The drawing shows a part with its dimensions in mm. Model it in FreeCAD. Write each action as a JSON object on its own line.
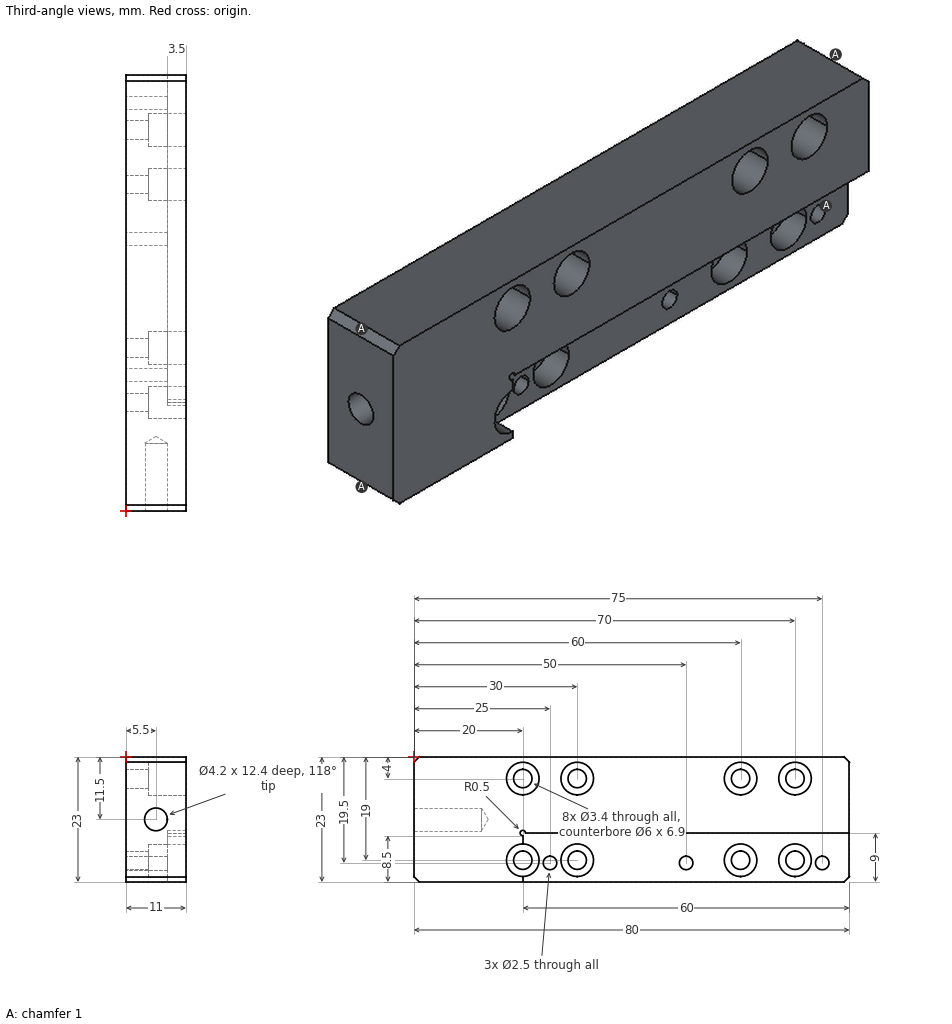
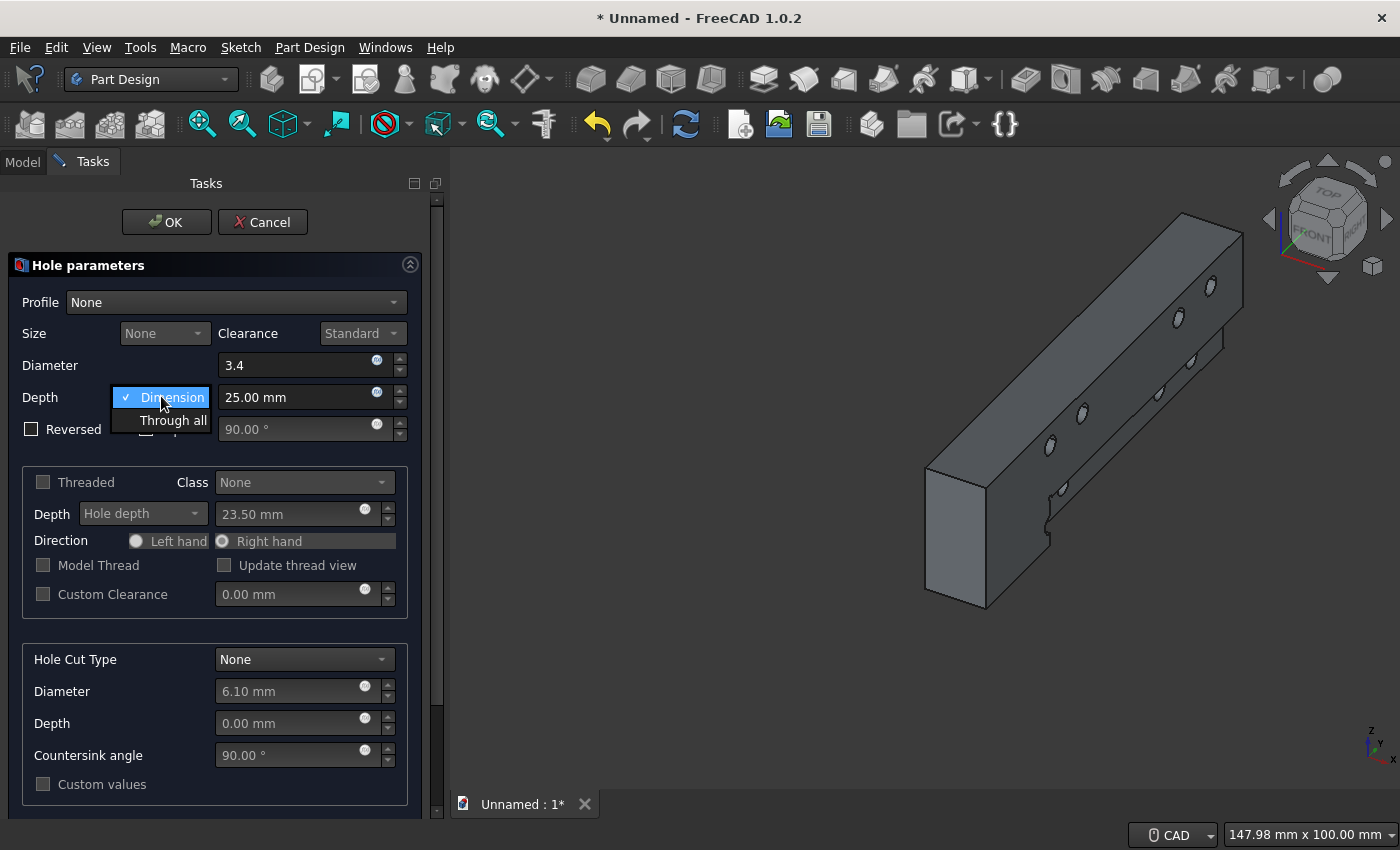
{"action": "left_click", "coordinate": [160, 420]}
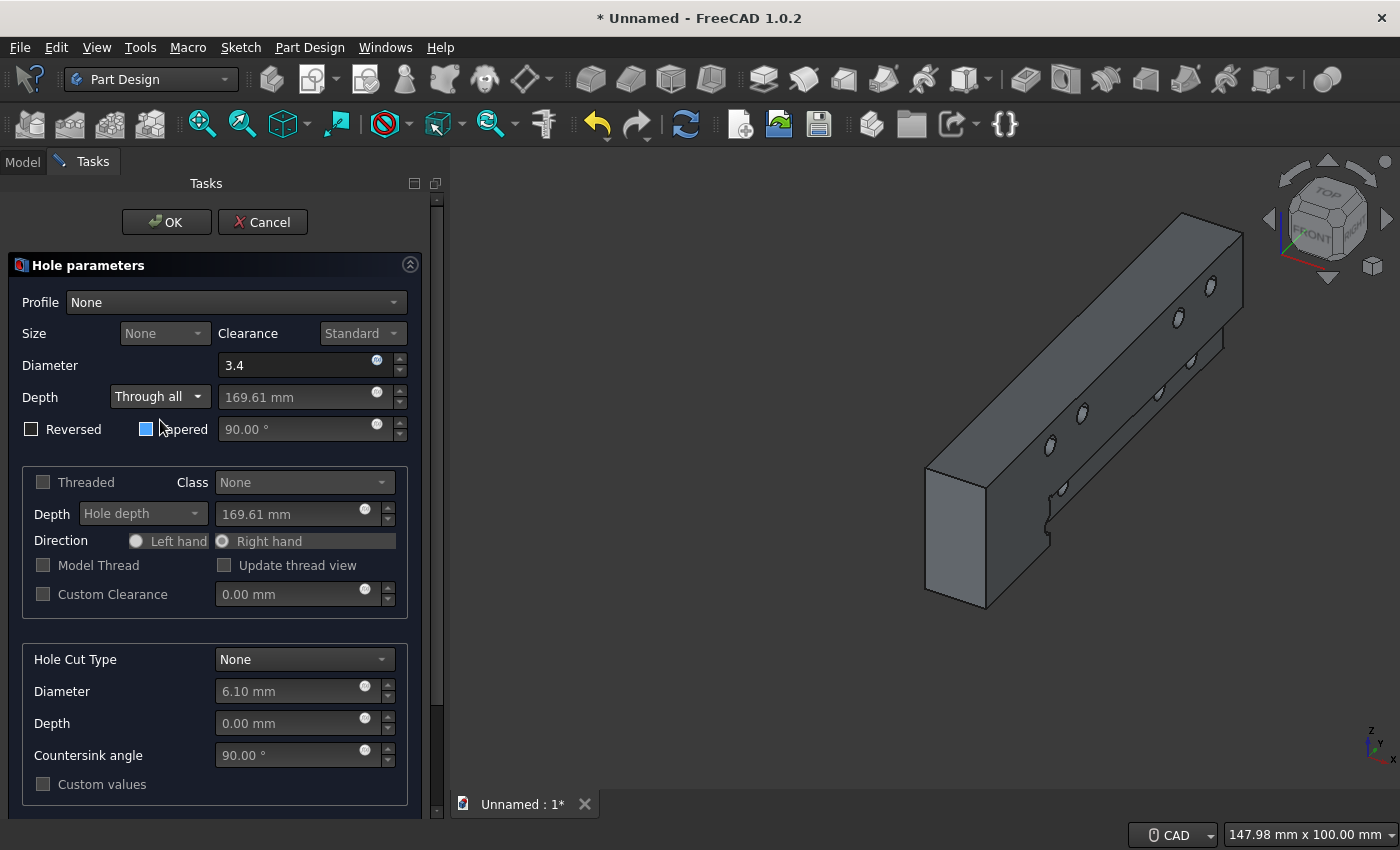
{"action": "left_click", "coordinate": [306, 660]}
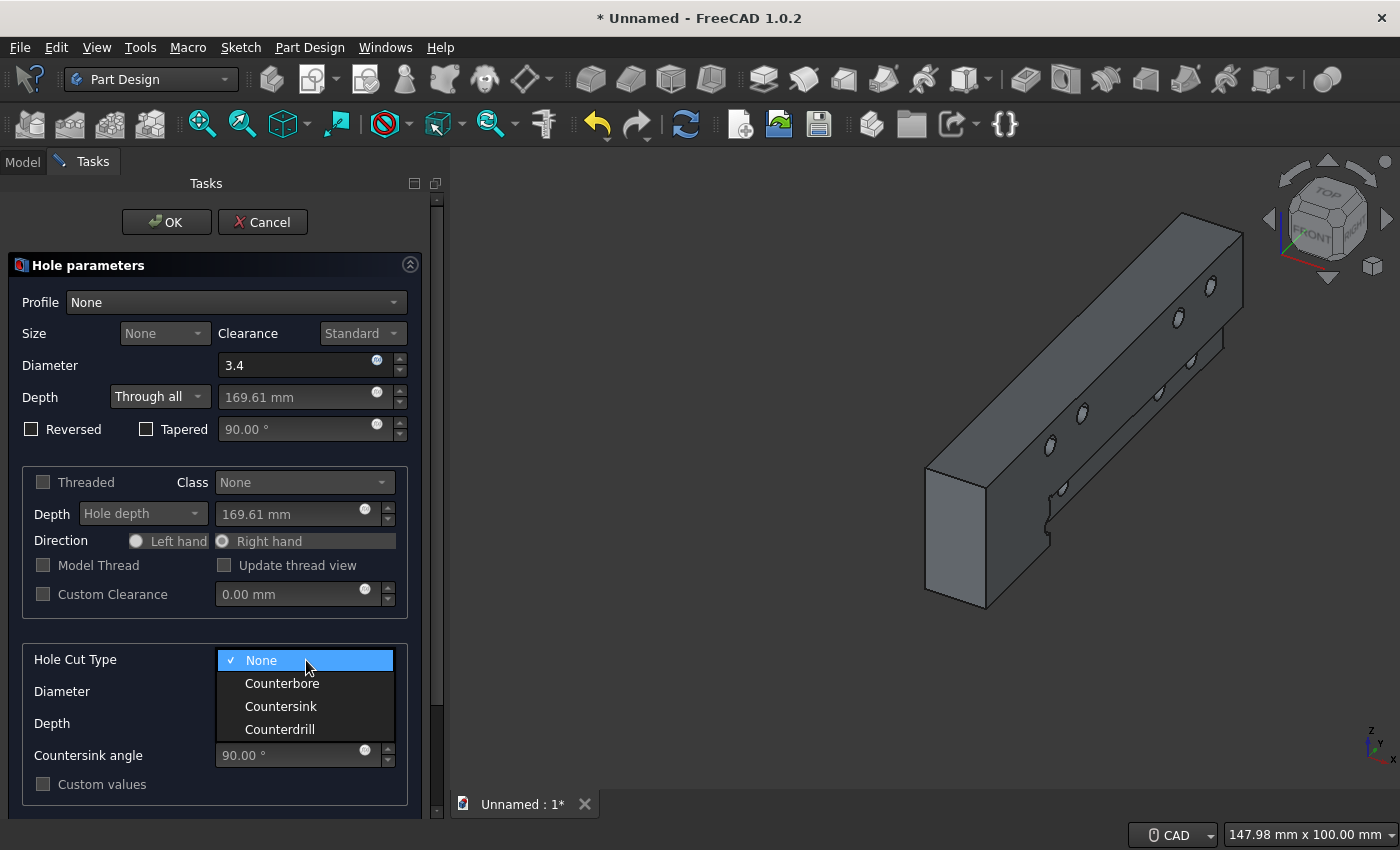
{"action": "left_click", "coordinate": [304, 684]}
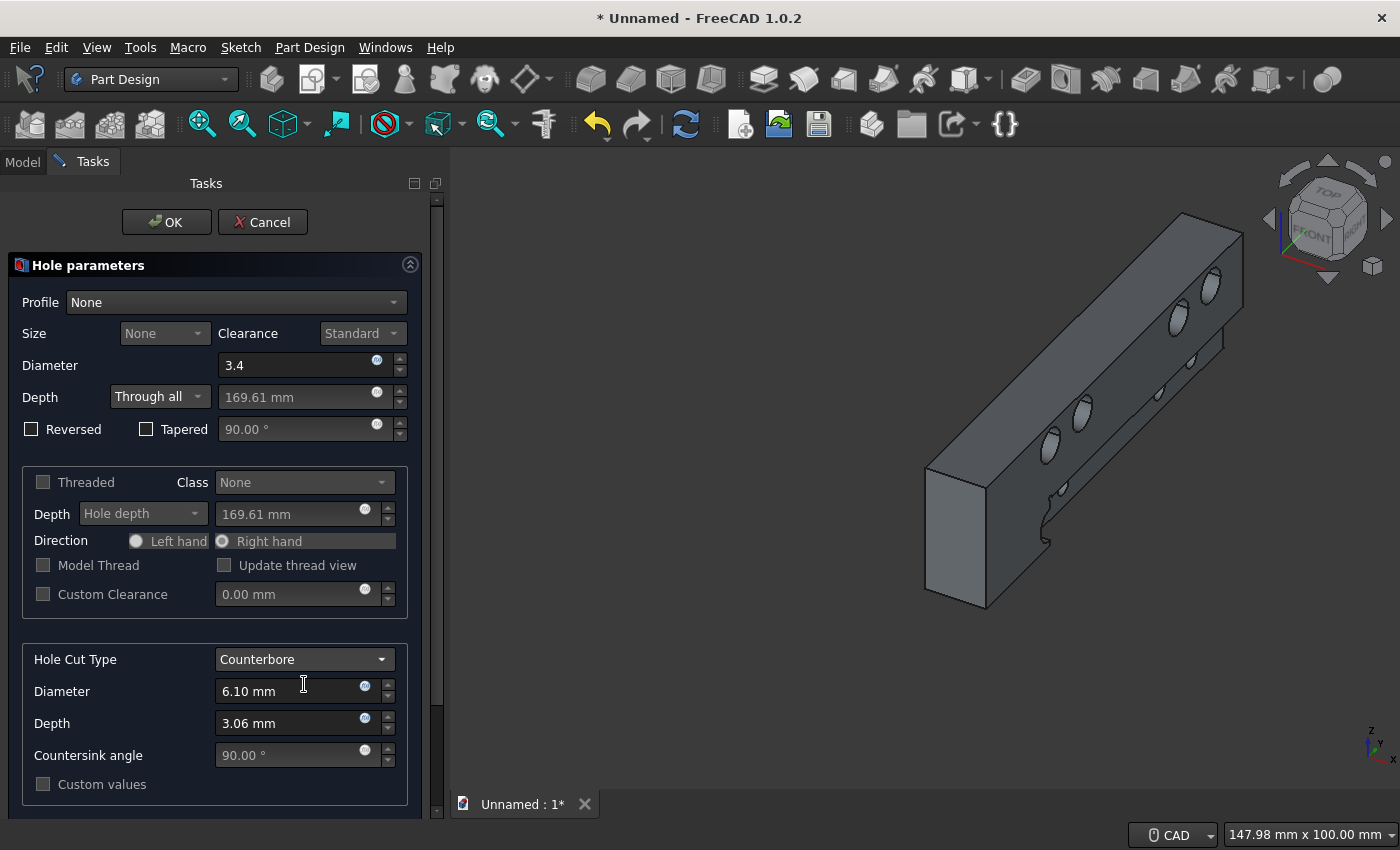
{"action": "triple_click", "coordinate": [298, 691]}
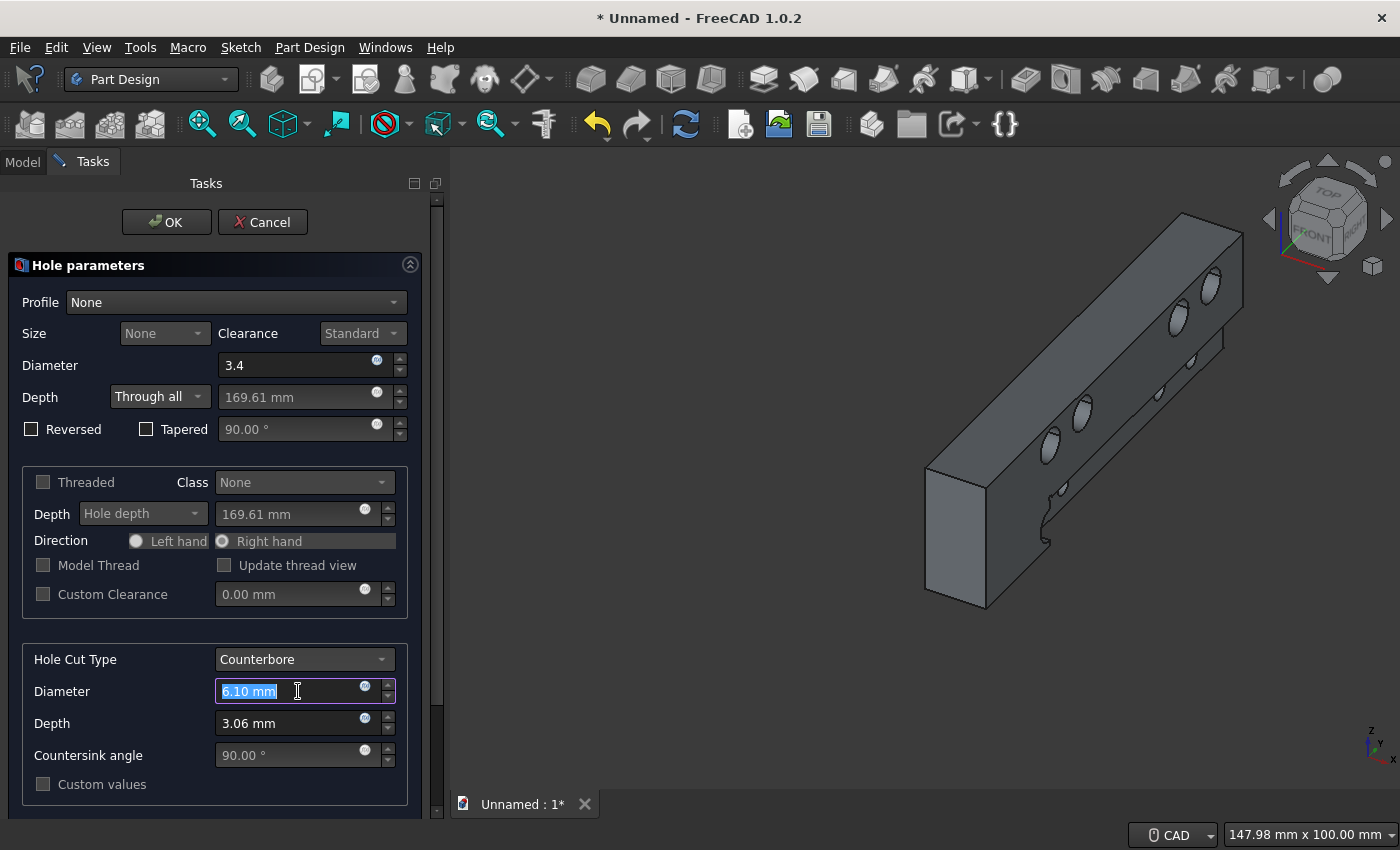
{"action": "type", "text": "6"}
{"action": "key", "text": "Tab"}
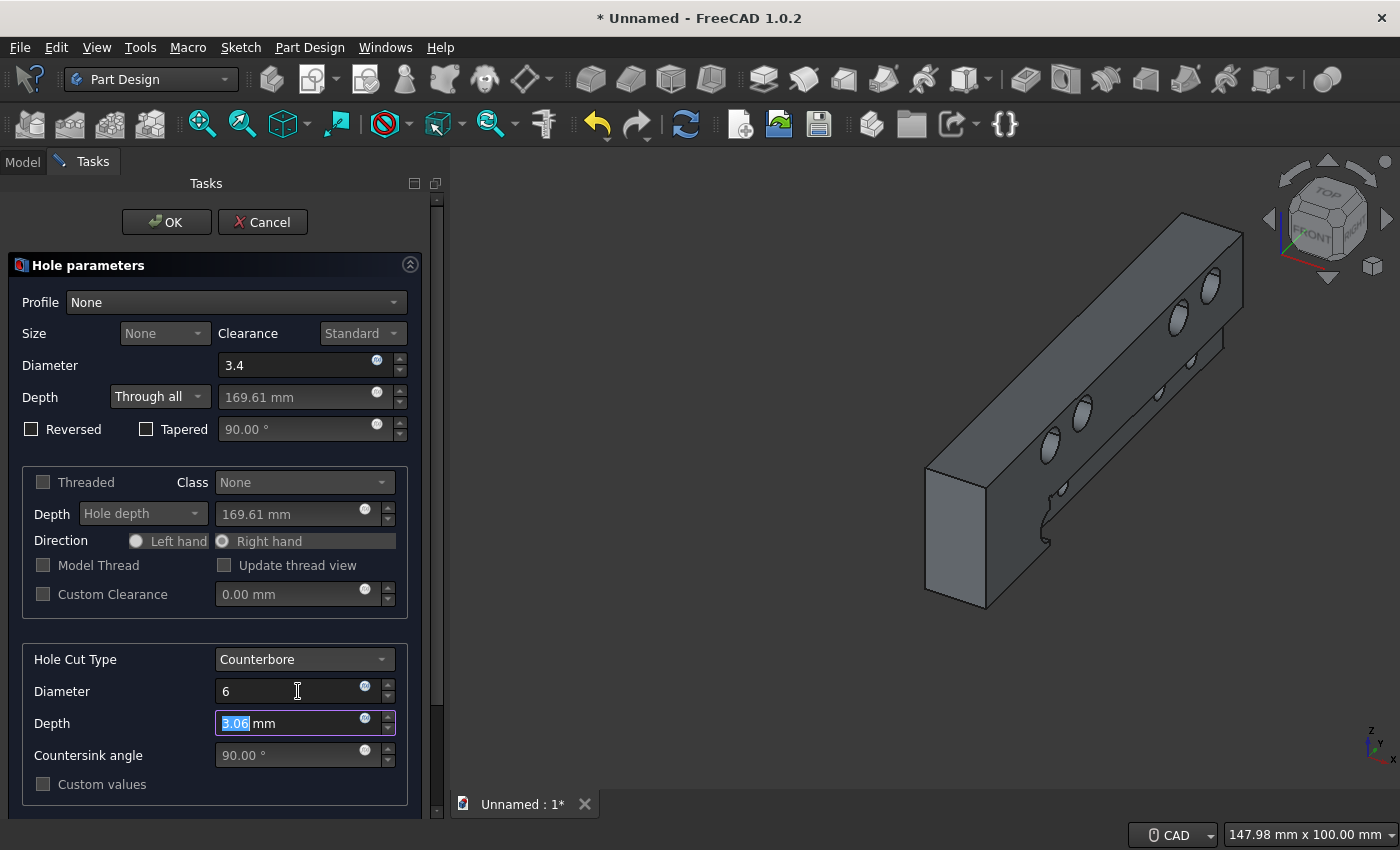
{"action": "type", "text": "6.9"}
{"action": "key", "text": "Tab"}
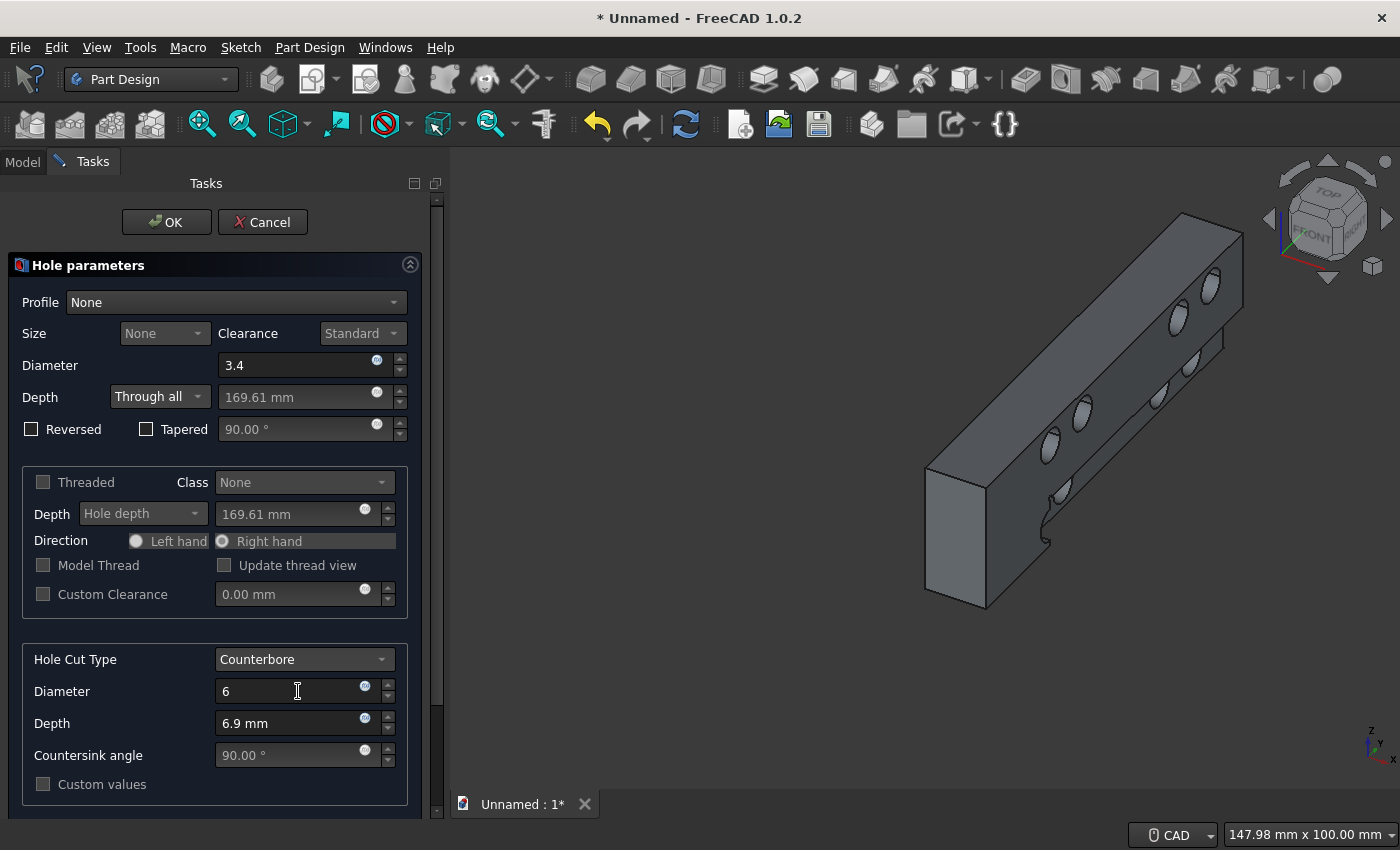
{"action": "left_click", "coordinate": [167, 222]}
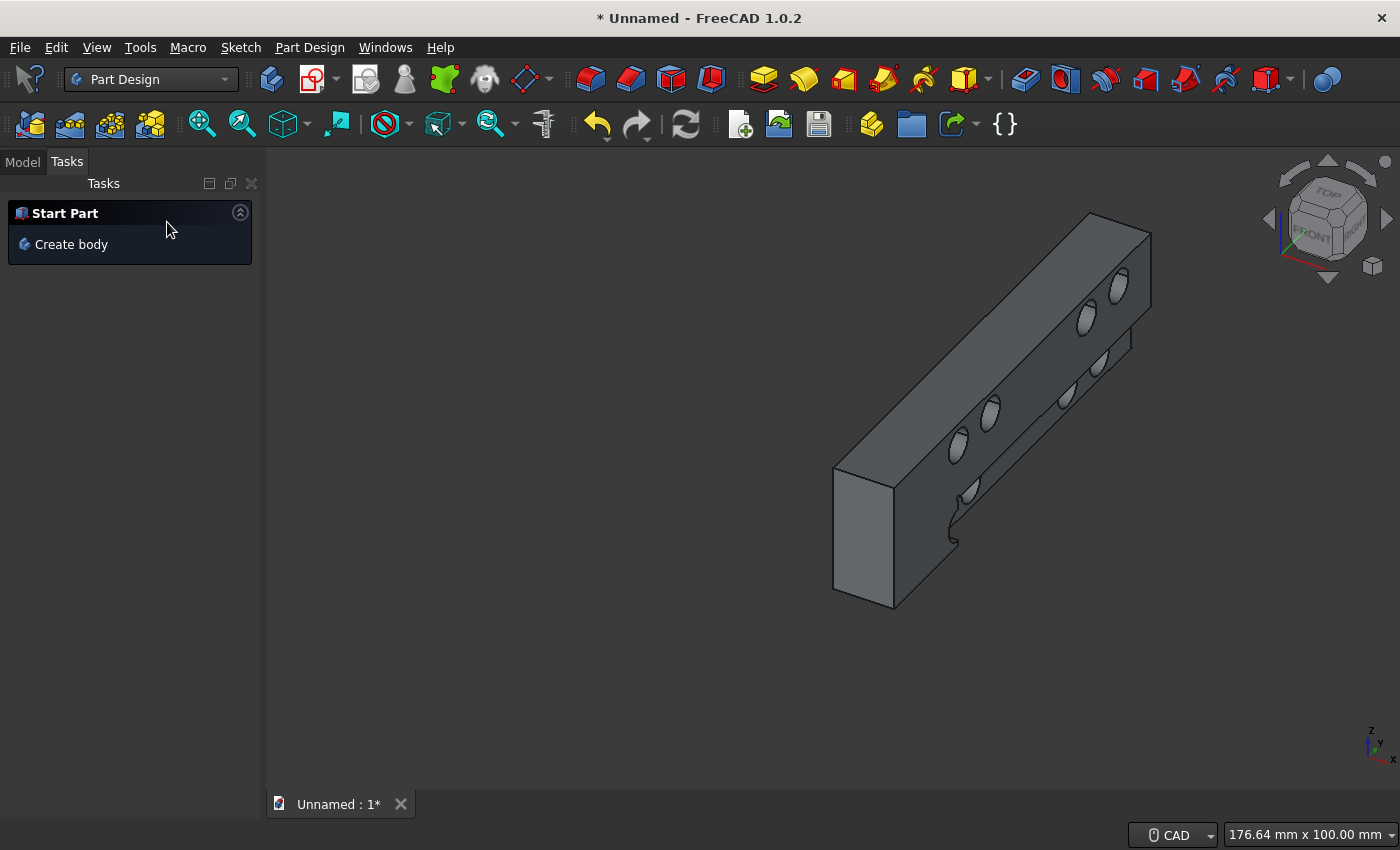
{"action": "left_click", "coordinate": [312, 80]}